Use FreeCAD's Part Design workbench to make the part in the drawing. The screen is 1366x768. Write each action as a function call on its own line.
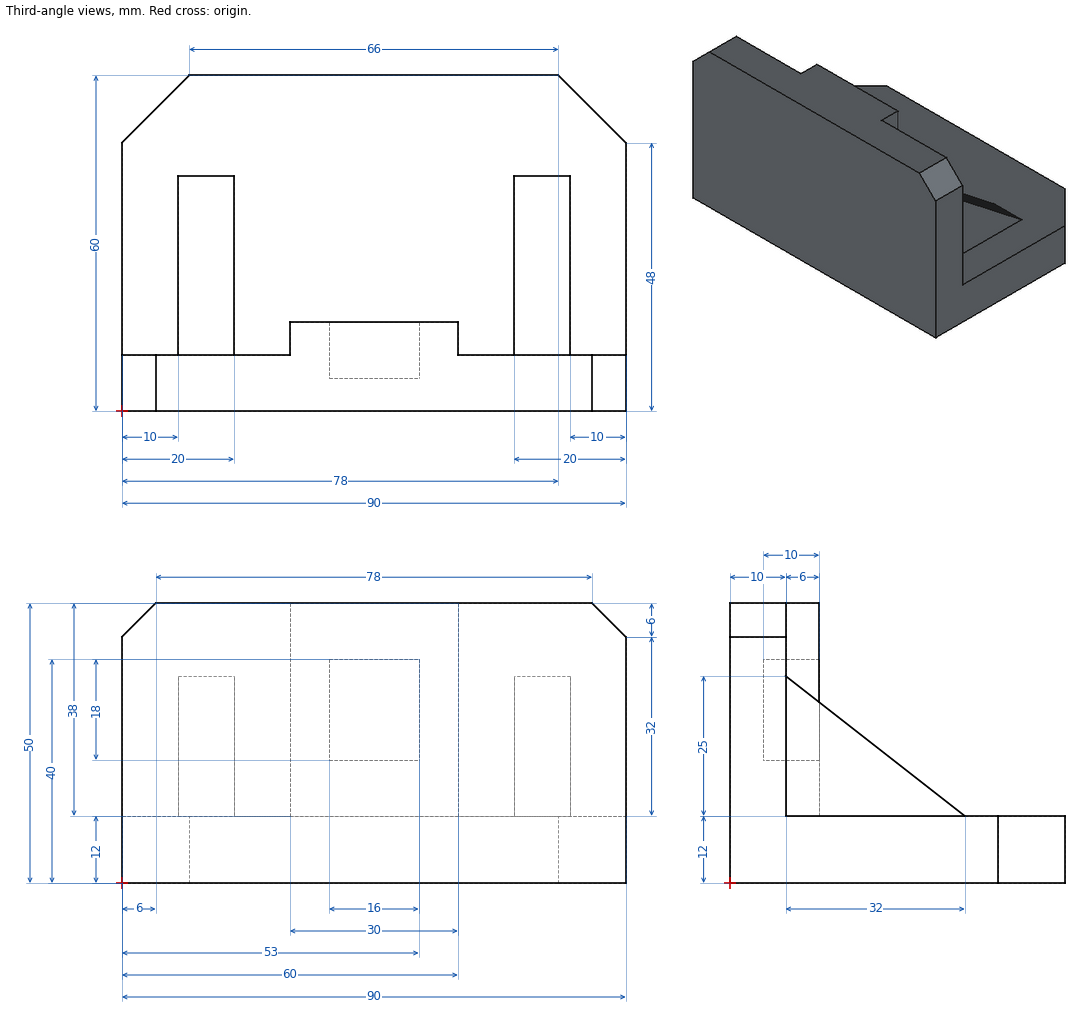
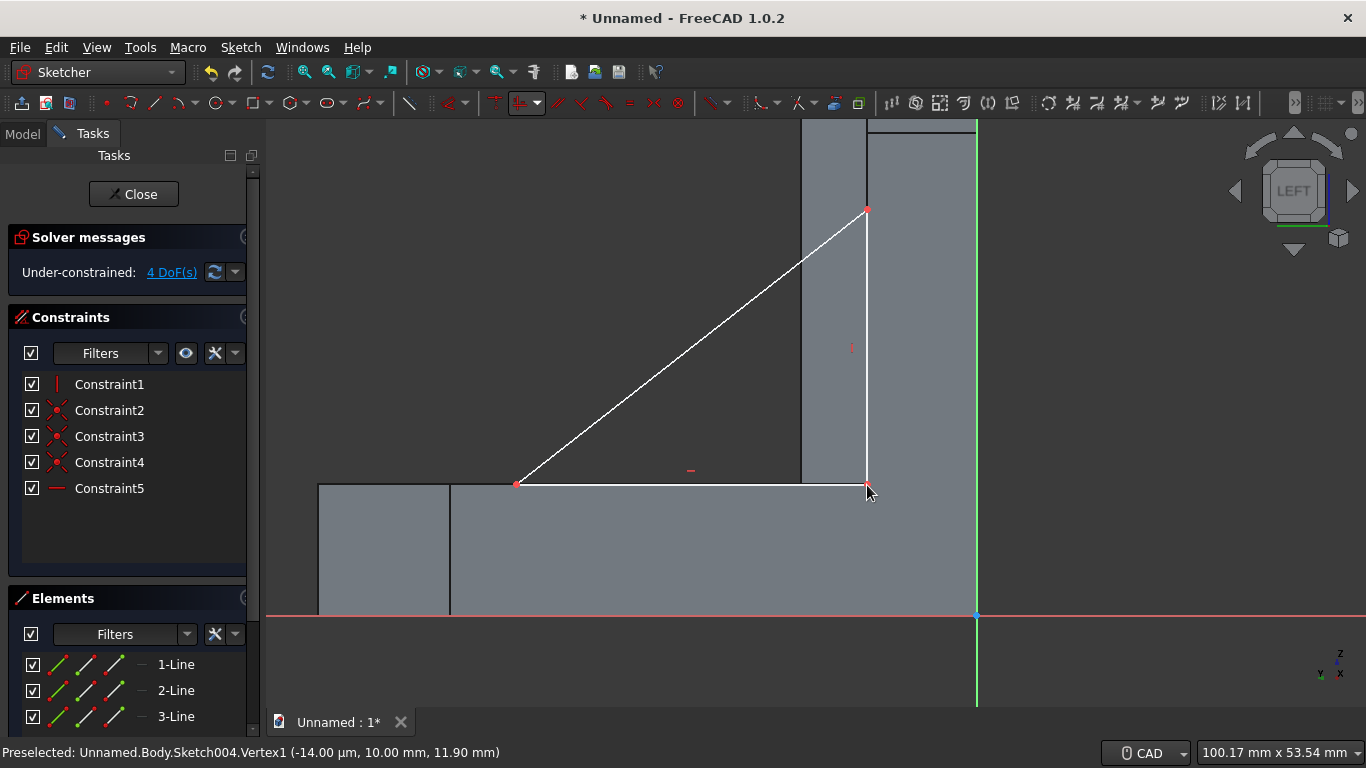
click(448, 104)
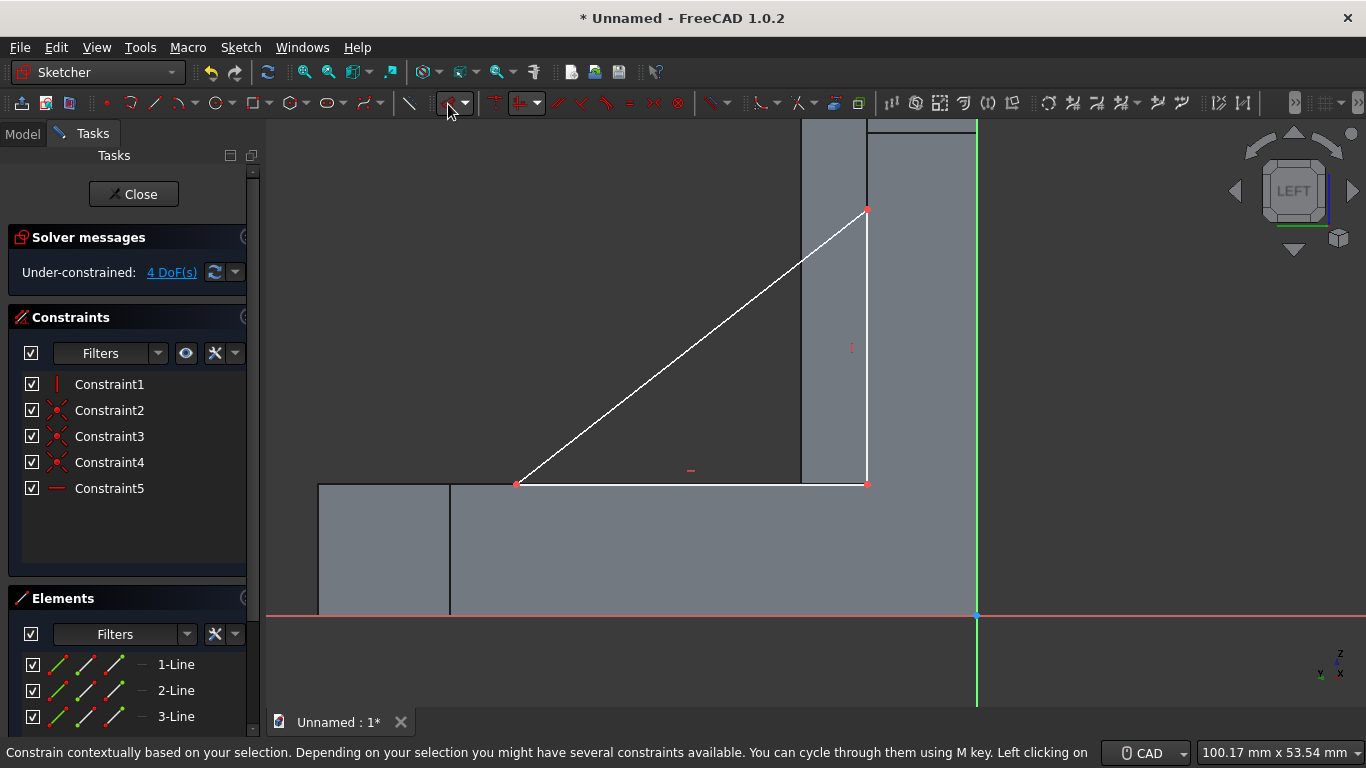
click(867, 403)
click(901, 347)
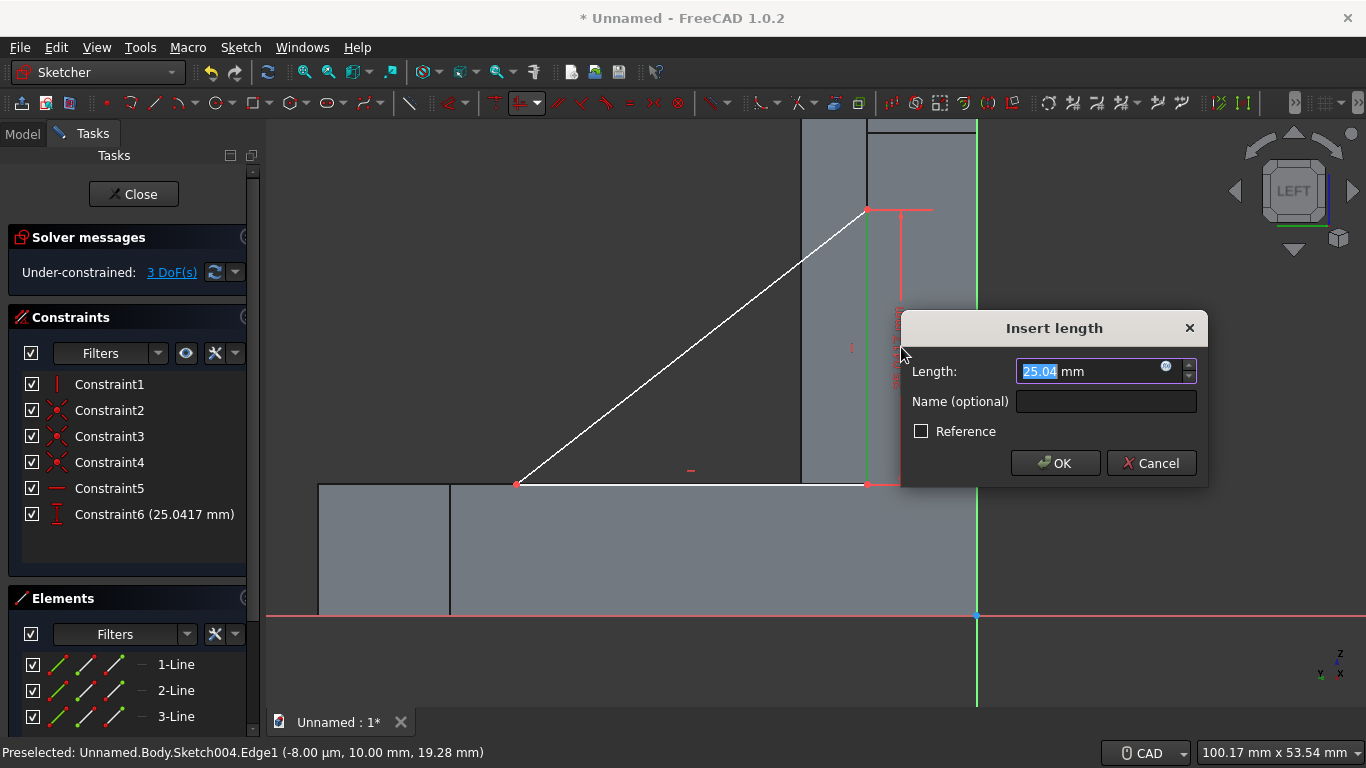
text(25)
key(Return)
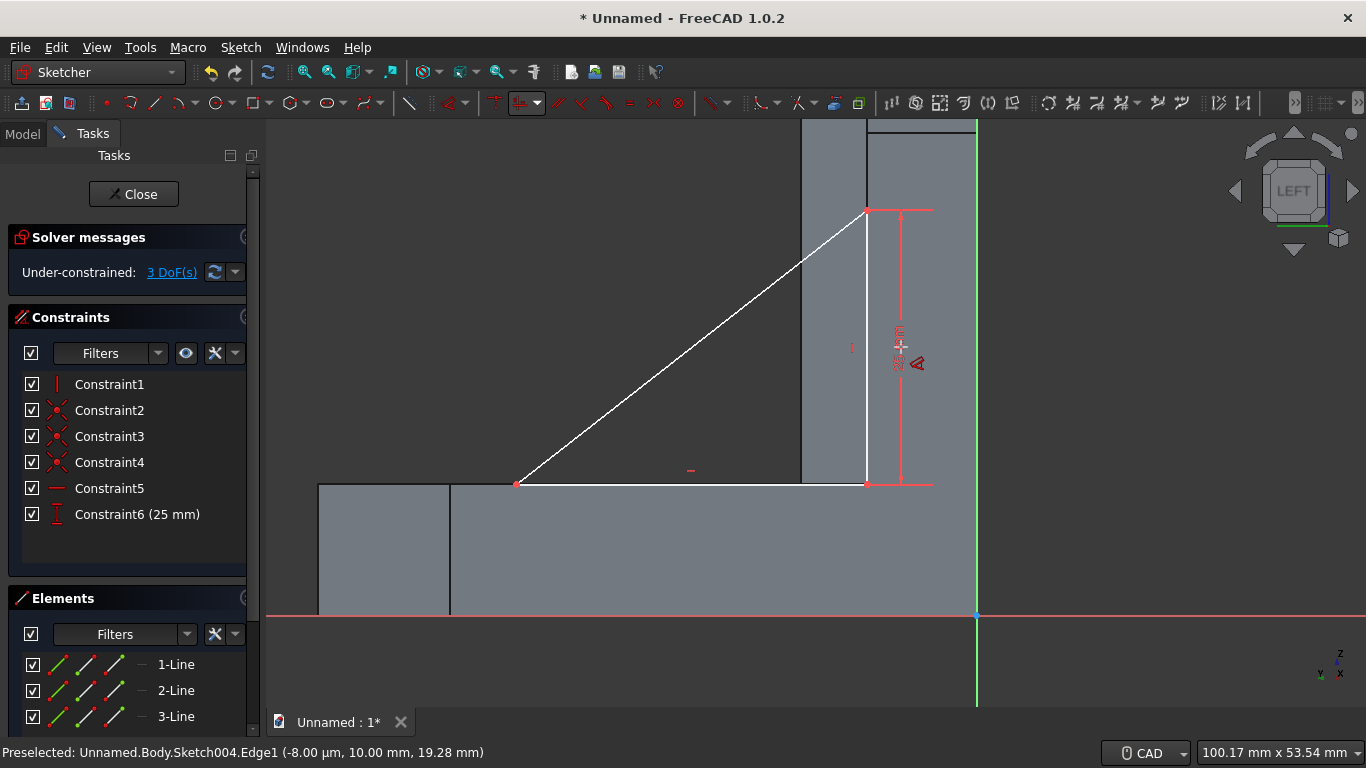
click(621, 485)
click(692, 519)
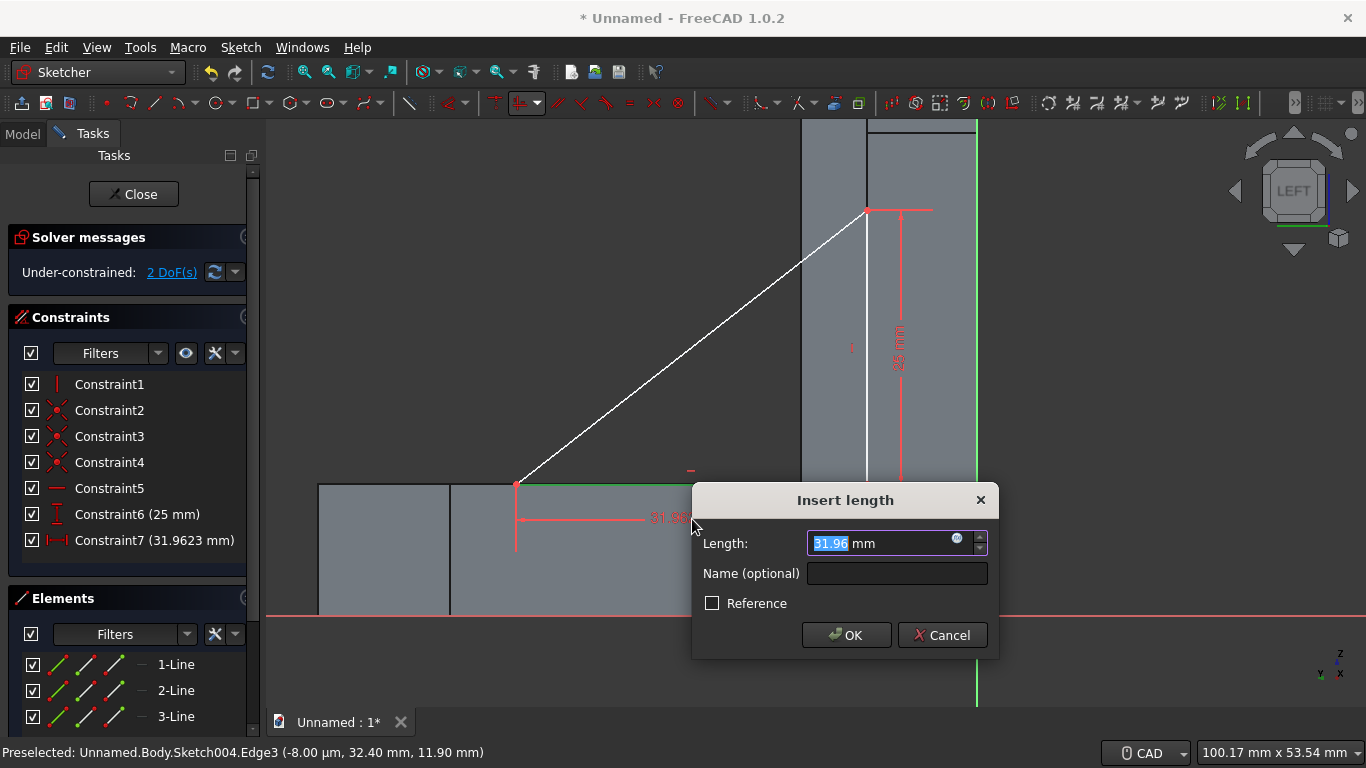
text(32)
key(Return)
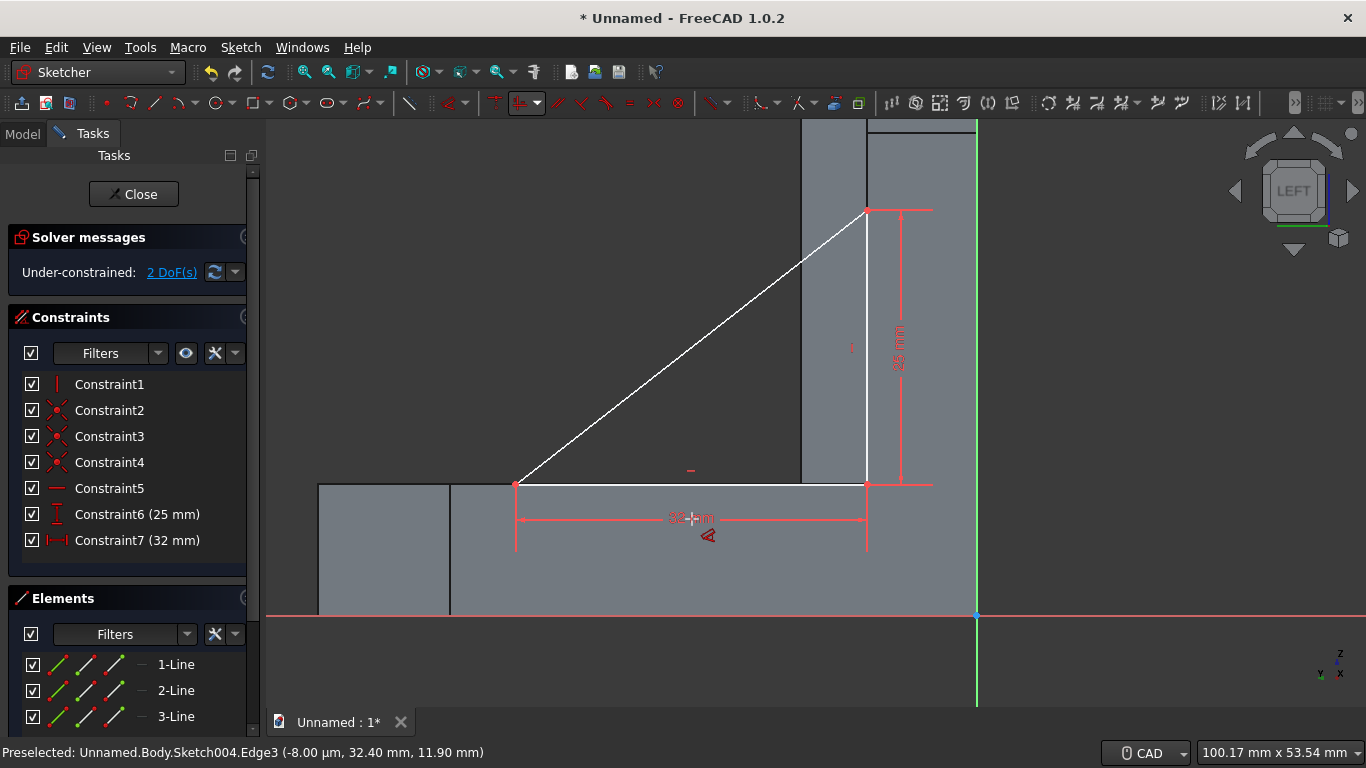
click(867, 485)
click(922, 650)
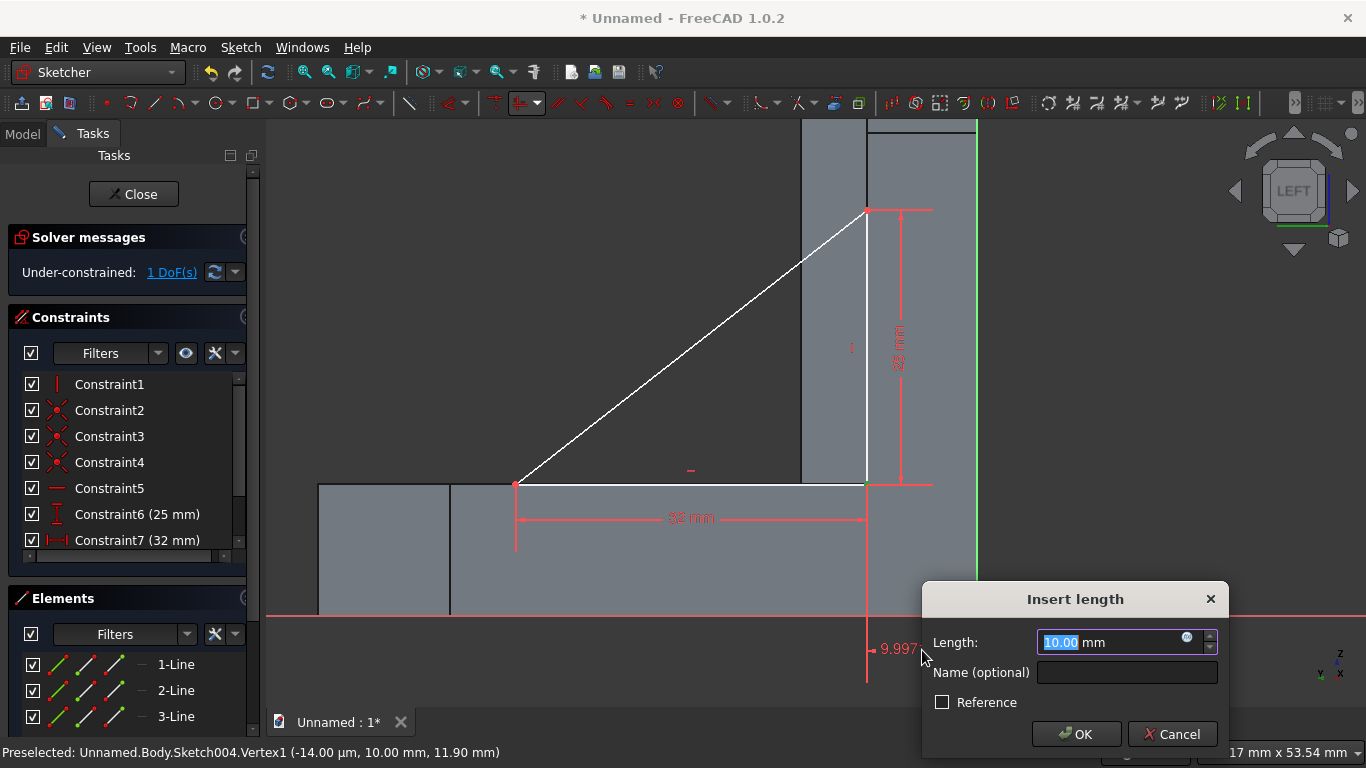
text(10)
key(Return)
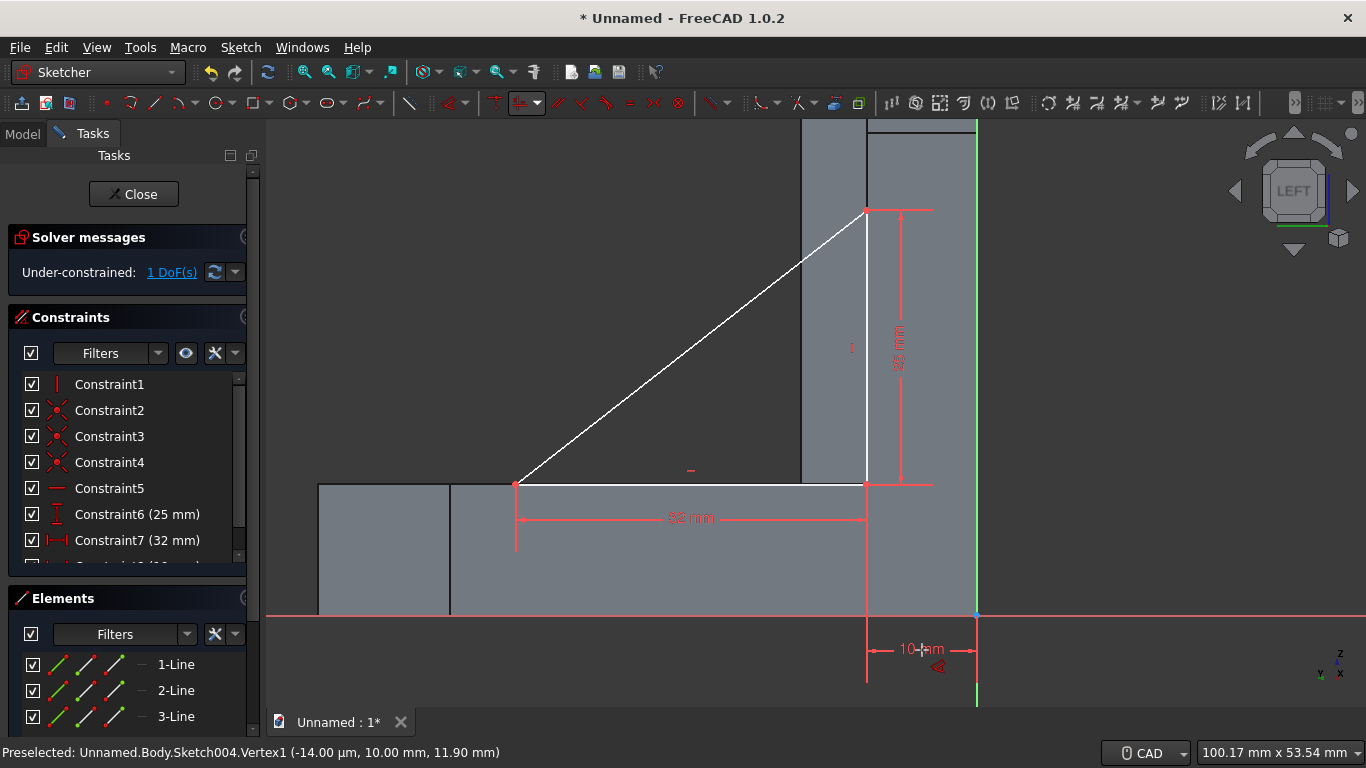
click(867, 485)
click(1011, 550)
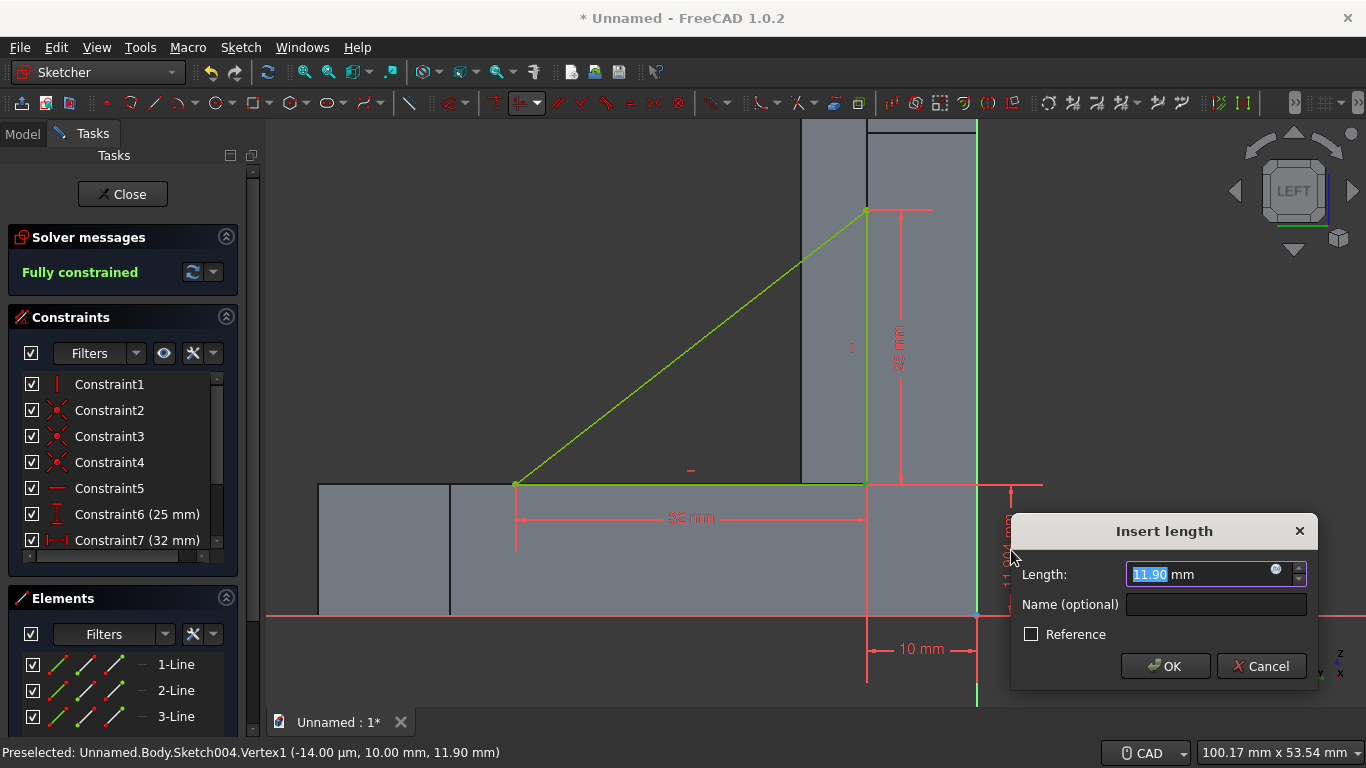
text(12)
key(Return)
key(Escape)